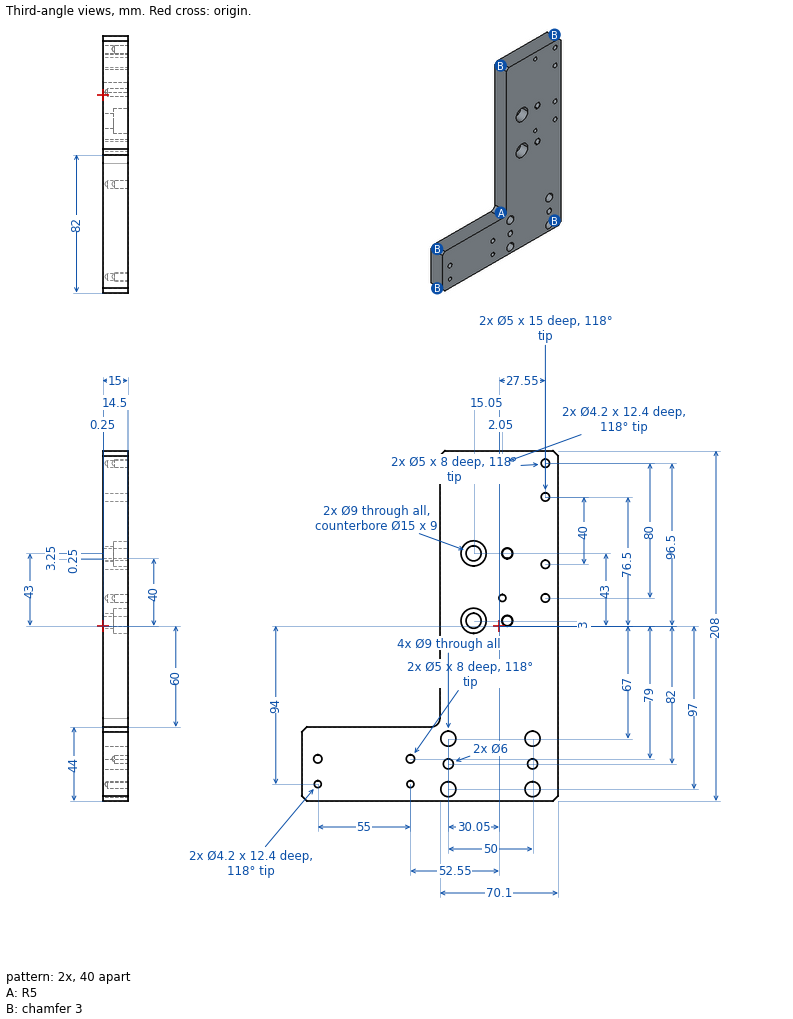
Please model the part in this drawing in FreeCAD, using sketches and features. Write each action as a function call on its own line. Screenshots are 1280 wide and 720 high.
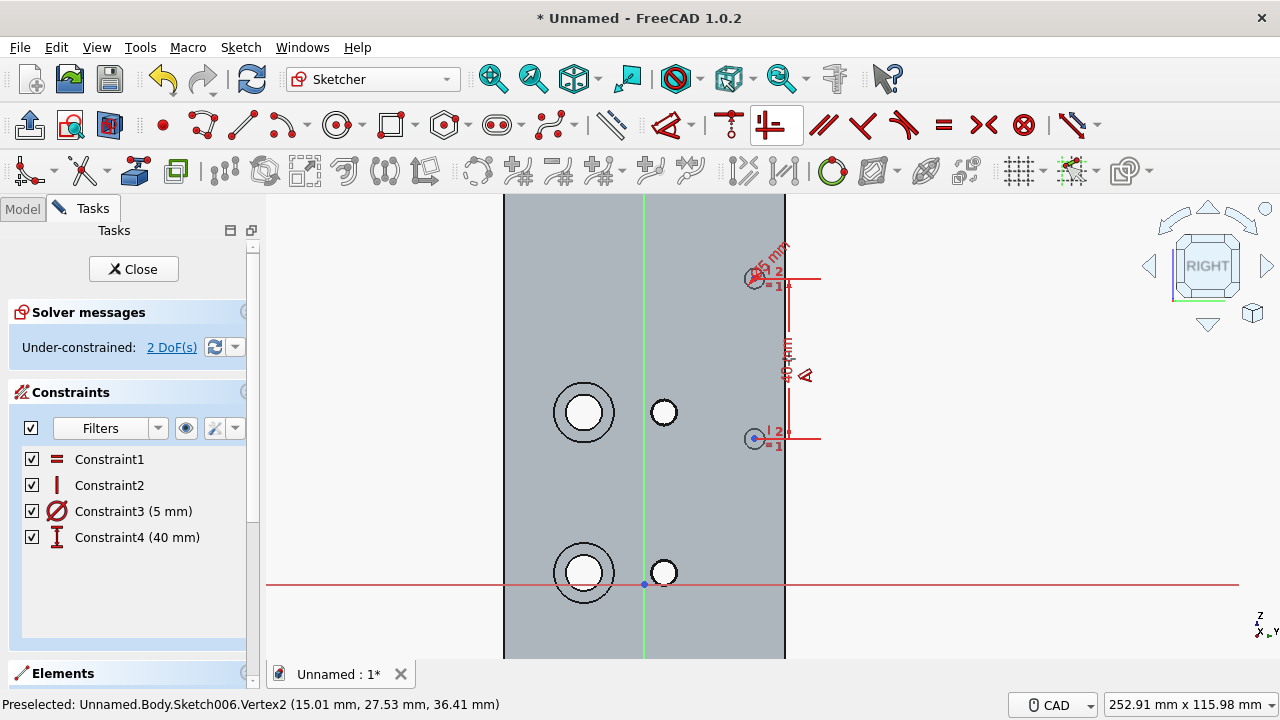
click(755, 279)
click(610, 432)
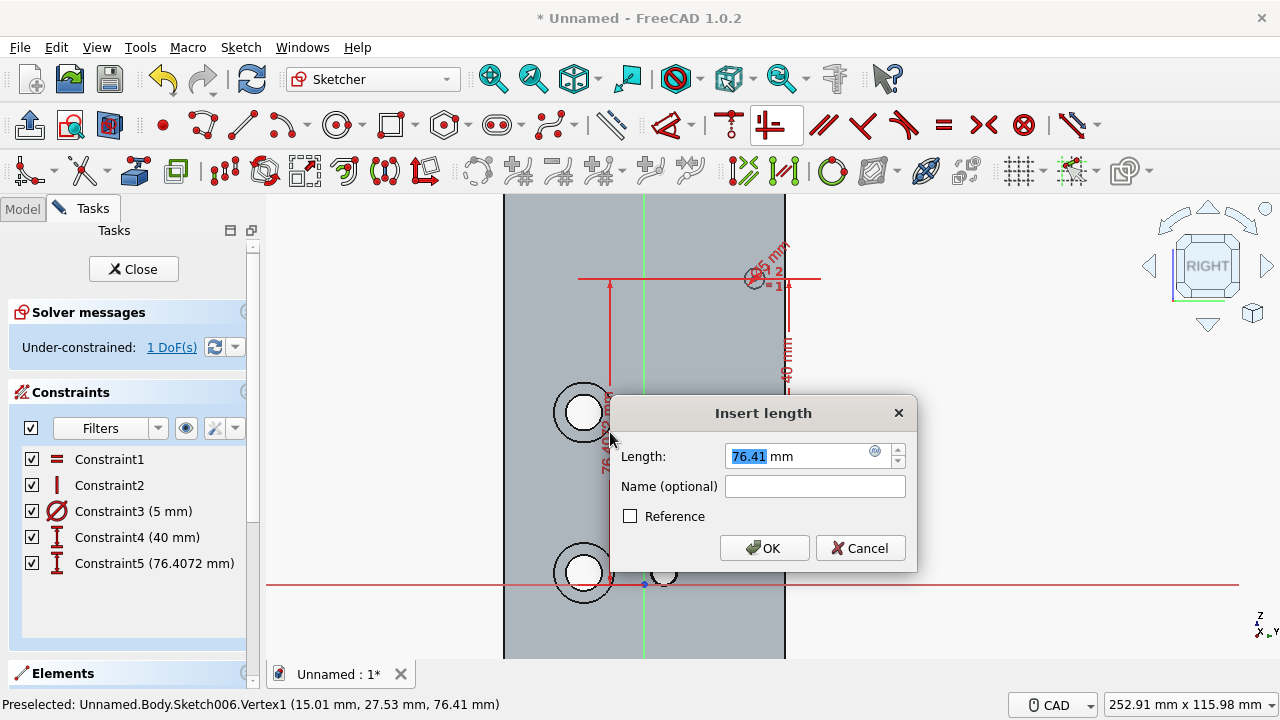
text(76.5)
key(Return)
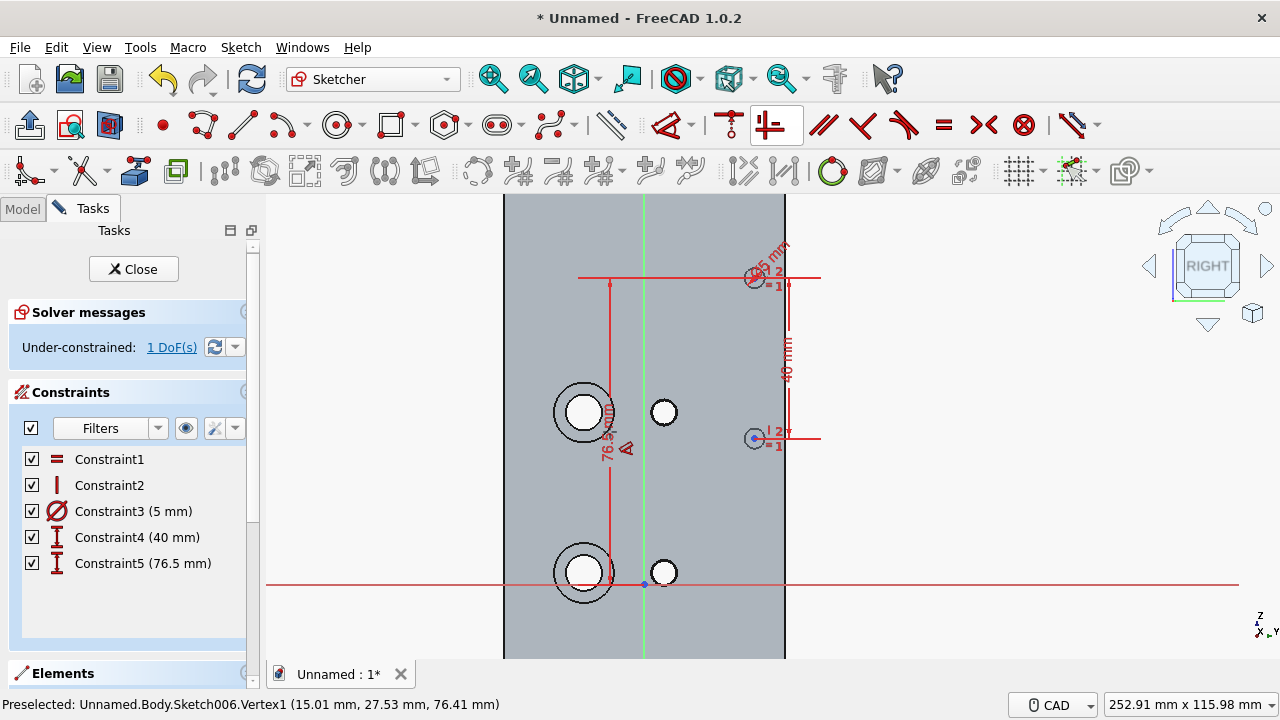
click(755, 278)
click(699, 619)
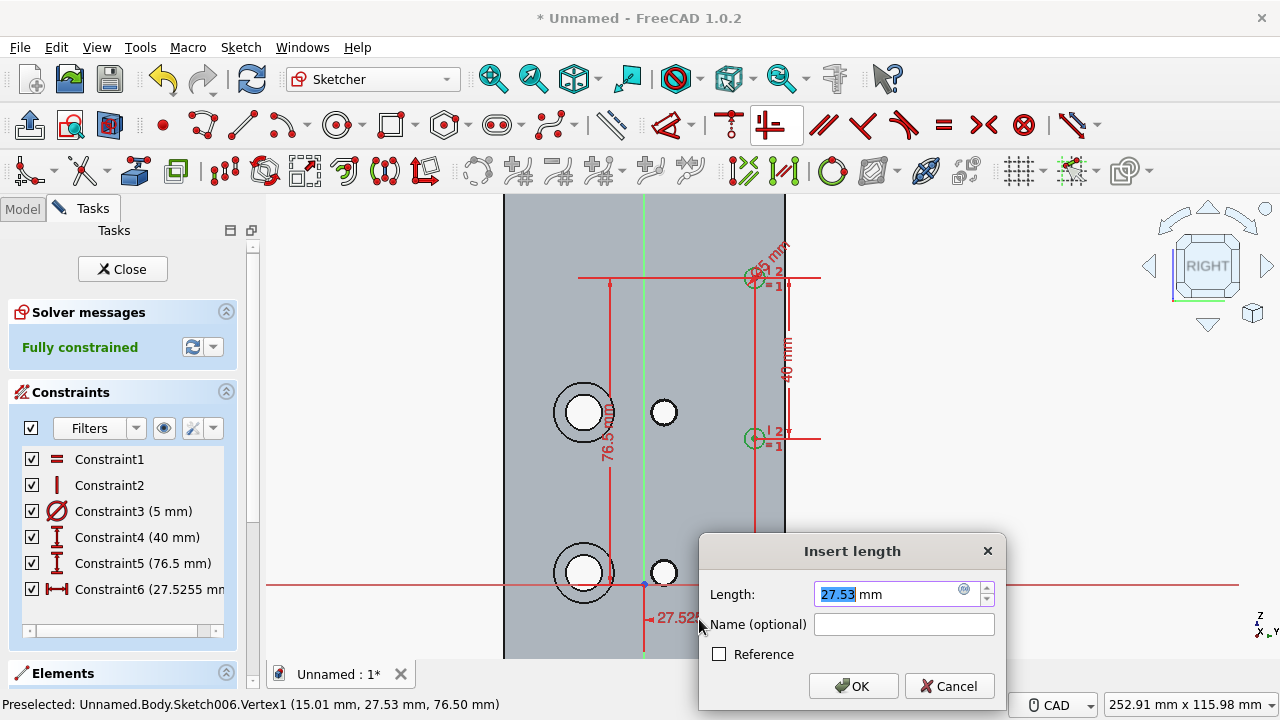
text(27.55)
key(Return)
key(Escape)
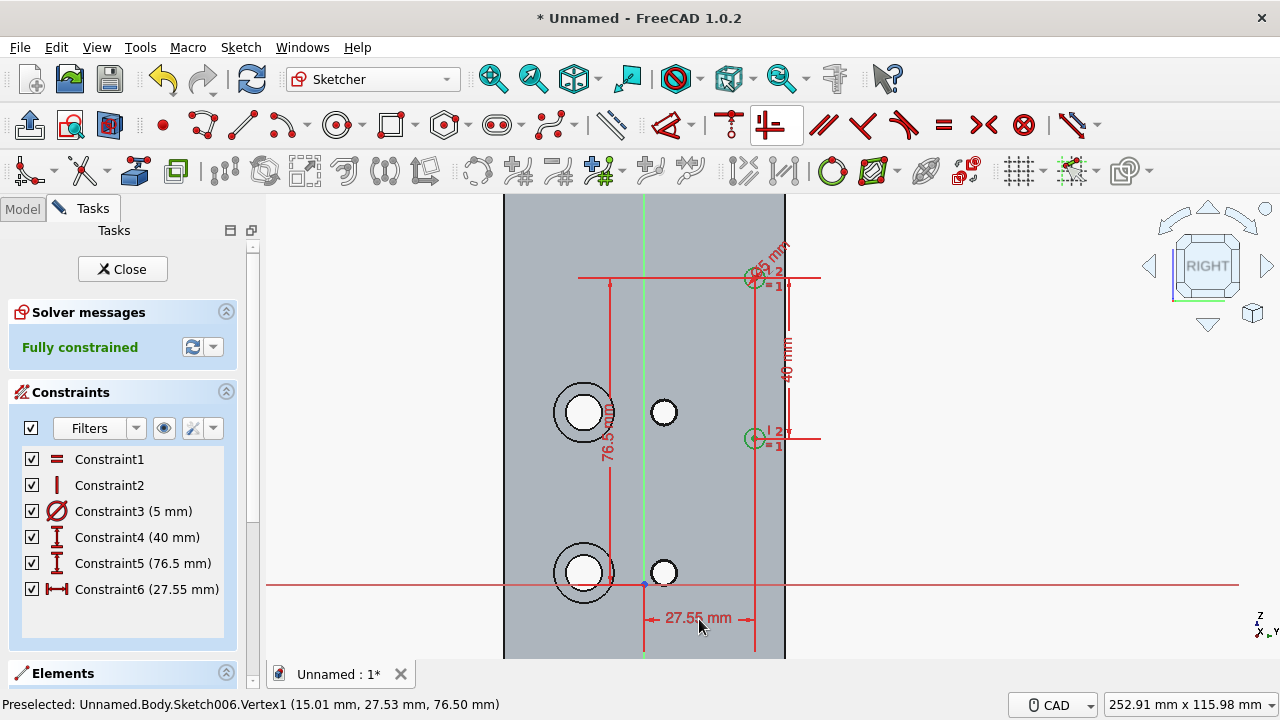
click(123, 269)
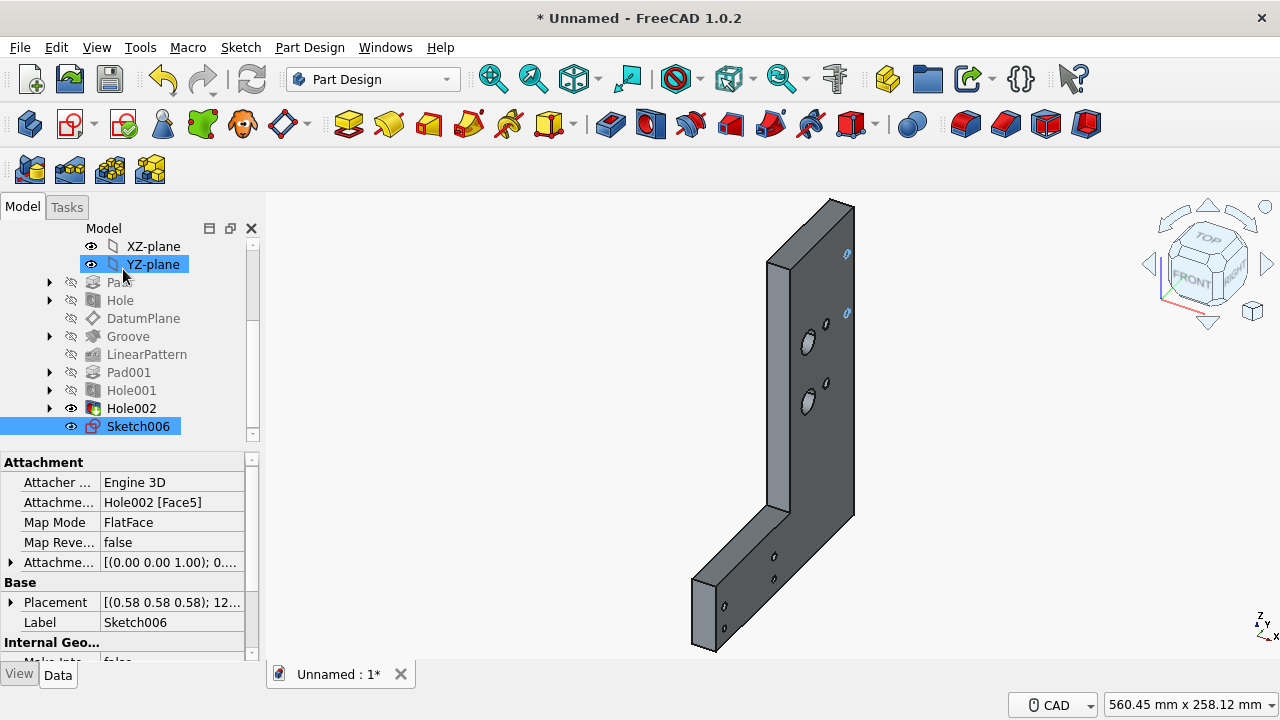
click(652, 124)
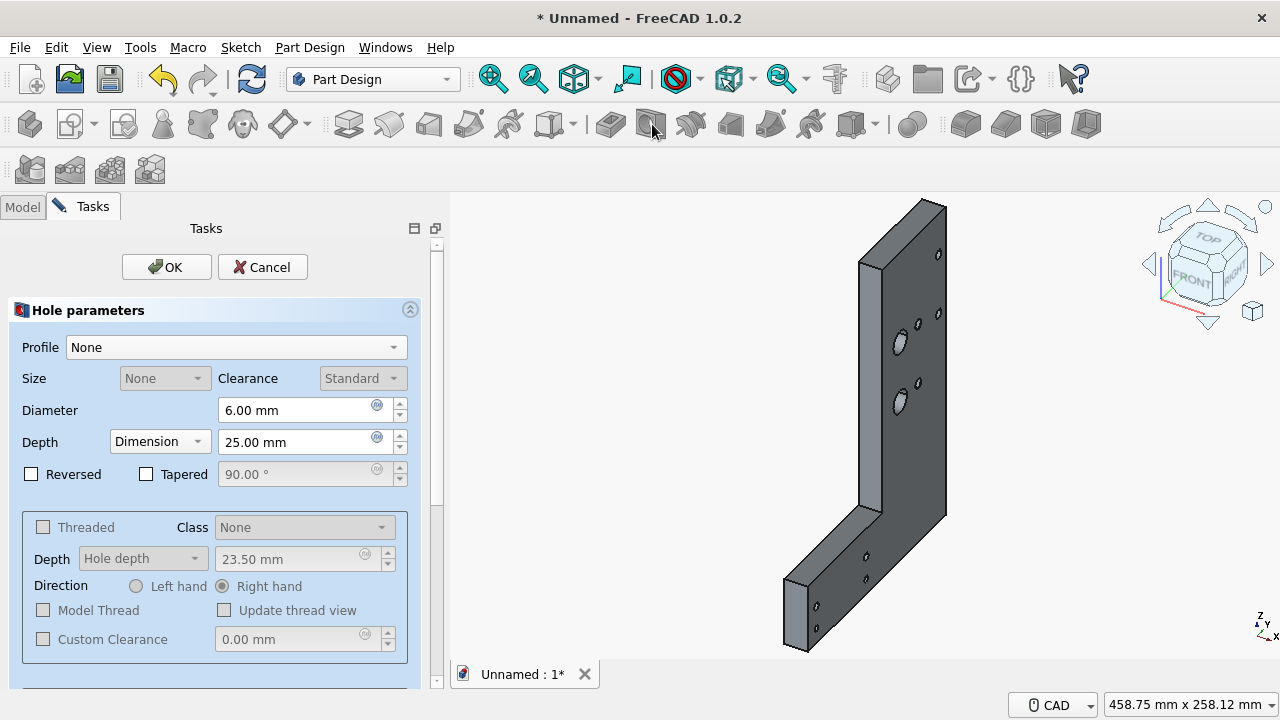
triple_click(305, 410)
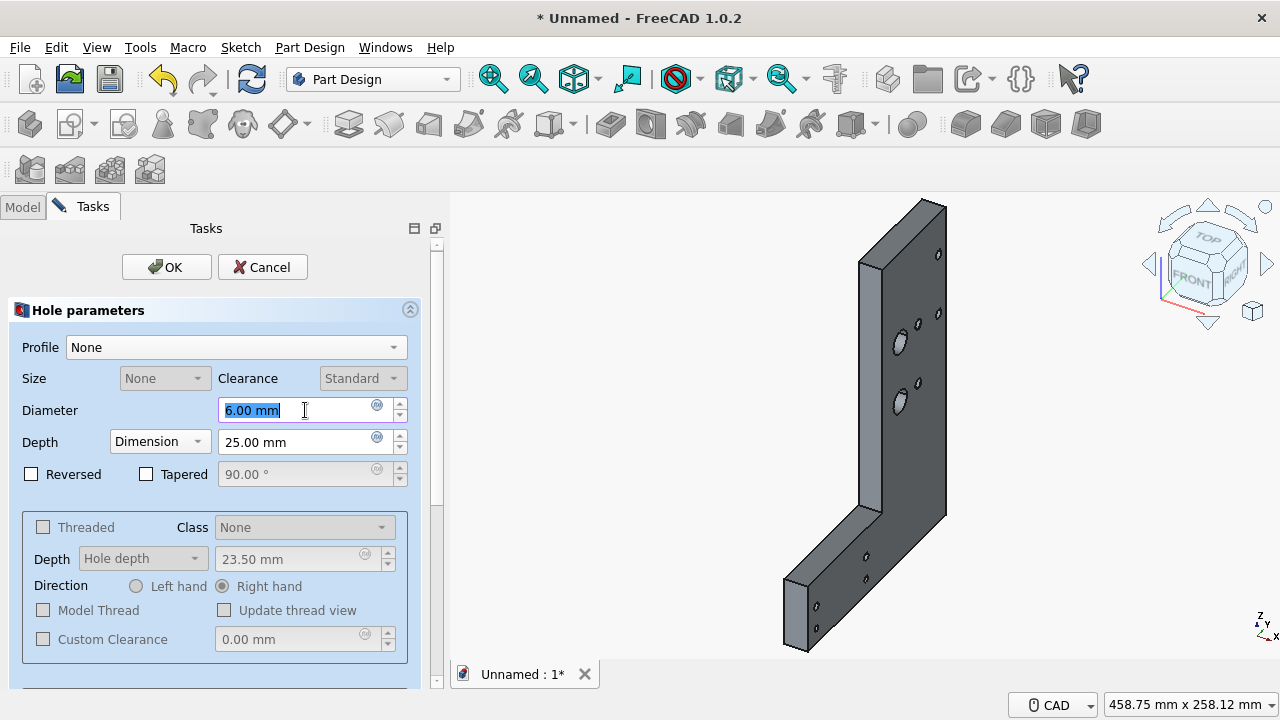
text(5)
key(Tab)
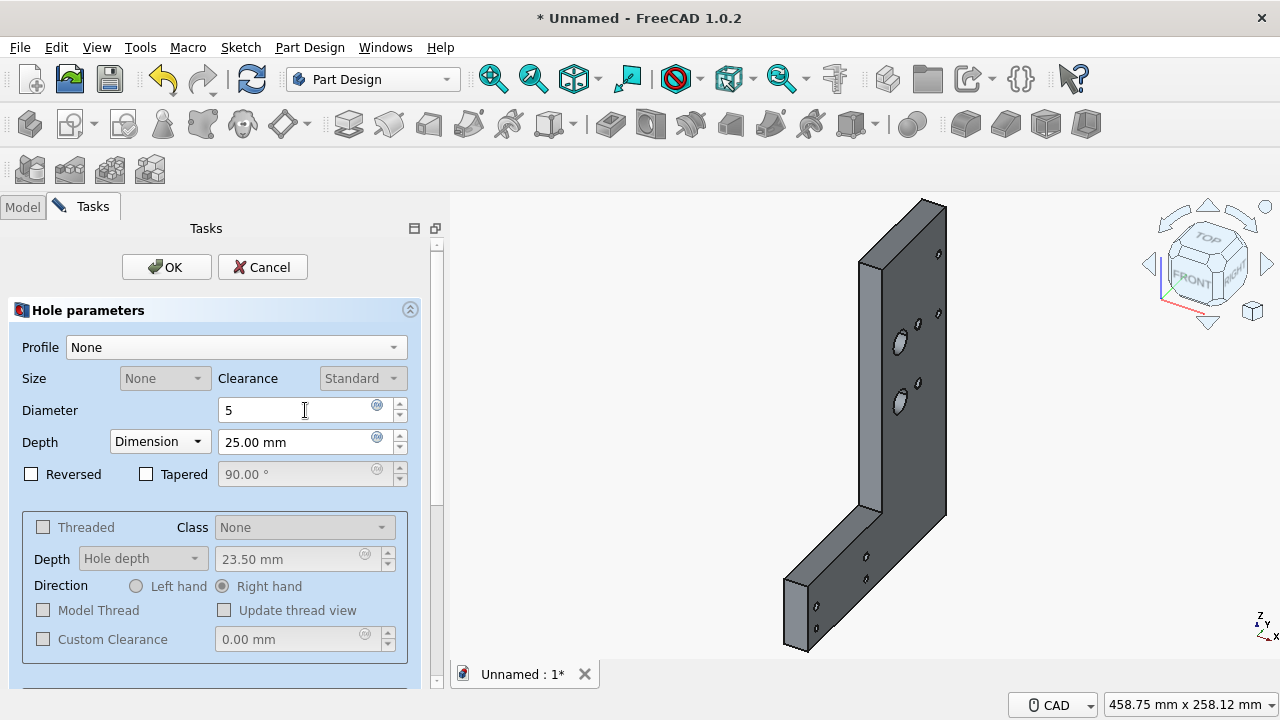
triple_click(305, 442)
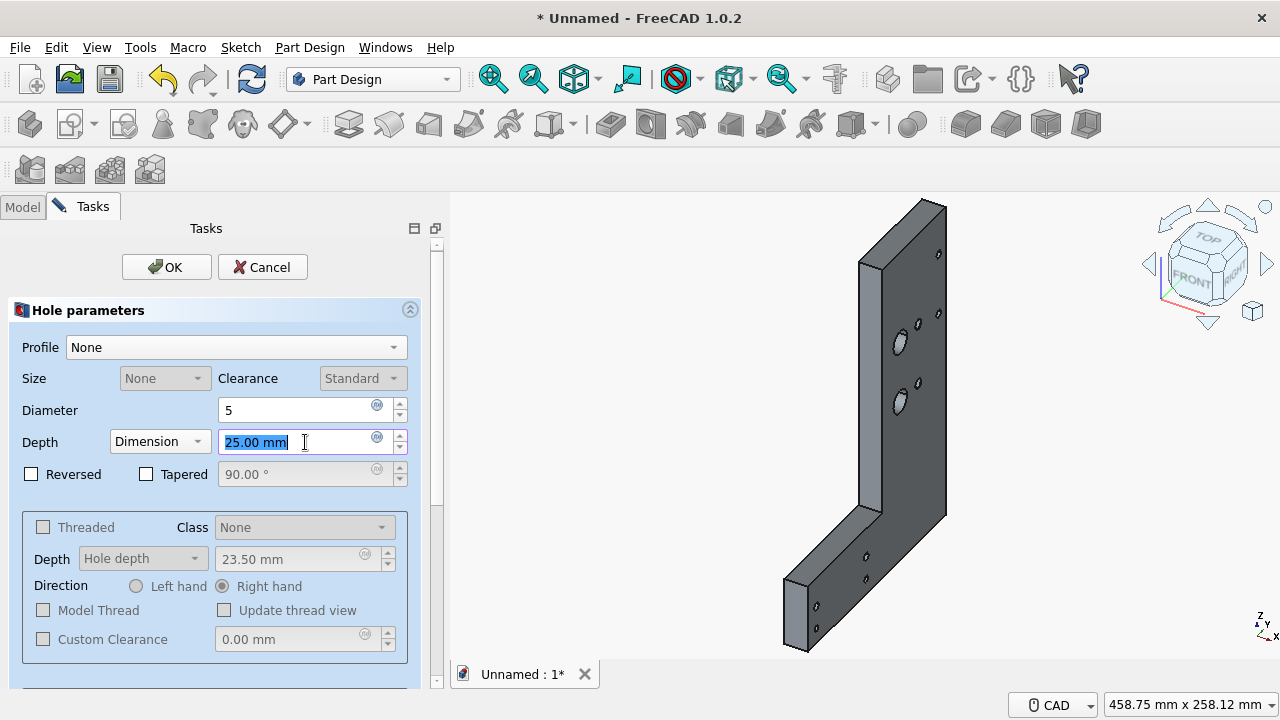
text(15)
key(Tab)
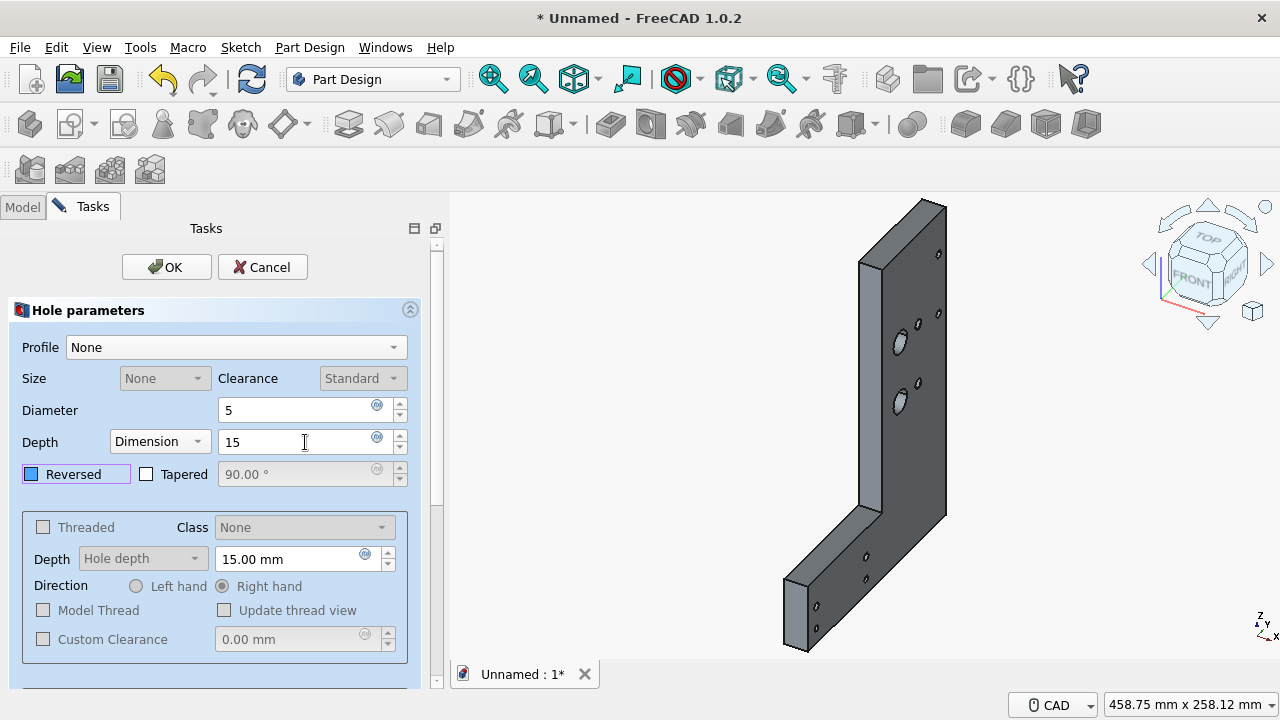
click(167, 267)